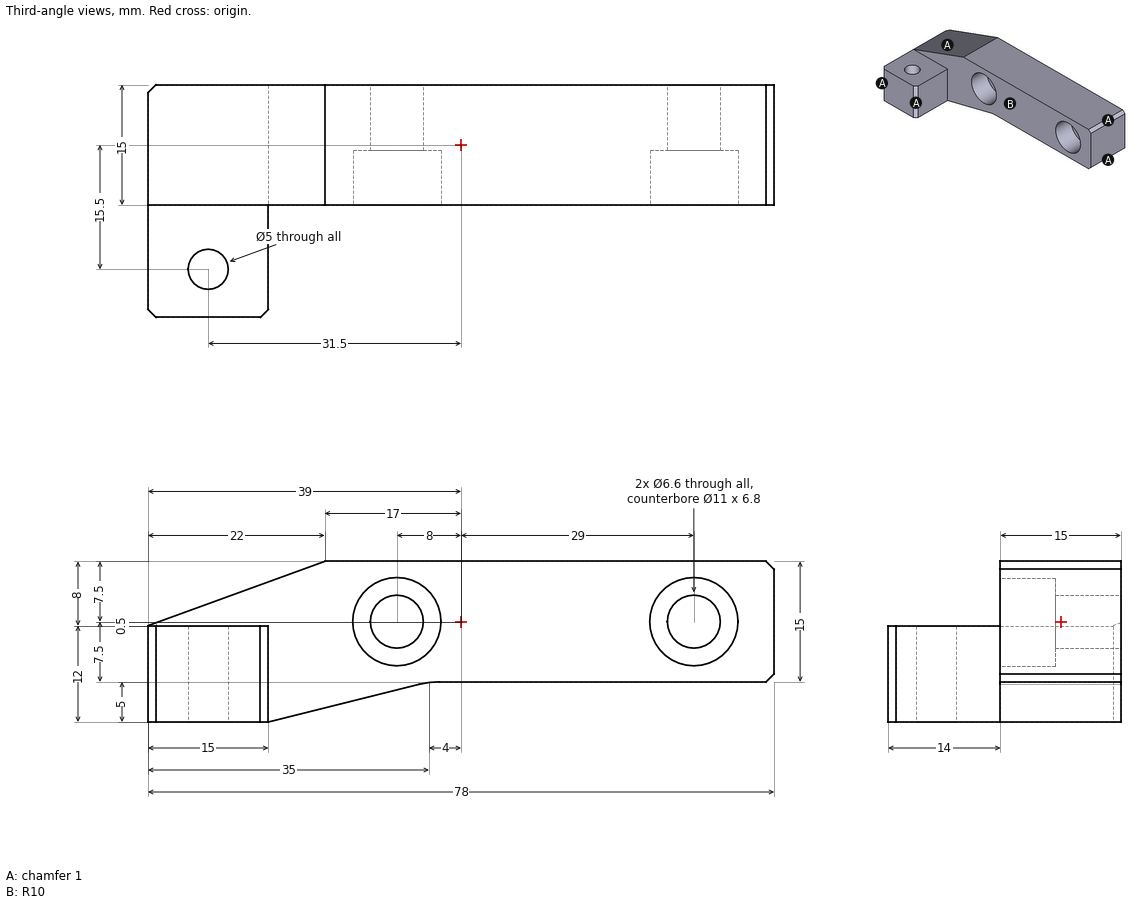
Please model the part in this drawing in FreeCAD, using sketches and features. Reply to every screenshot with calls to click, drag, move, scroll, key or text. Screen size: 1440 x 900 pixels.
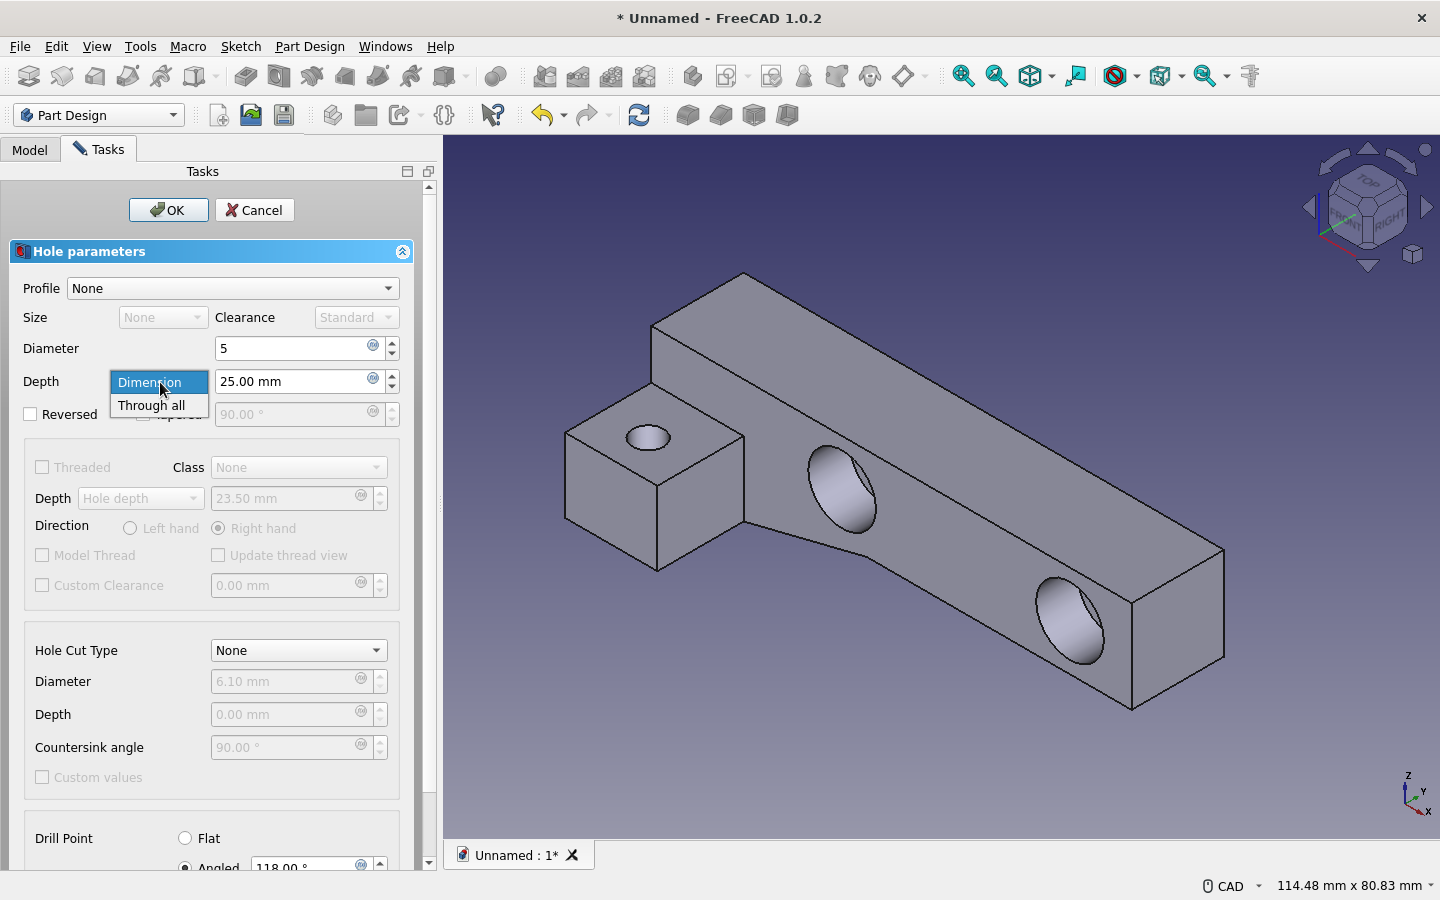
click(158, 406)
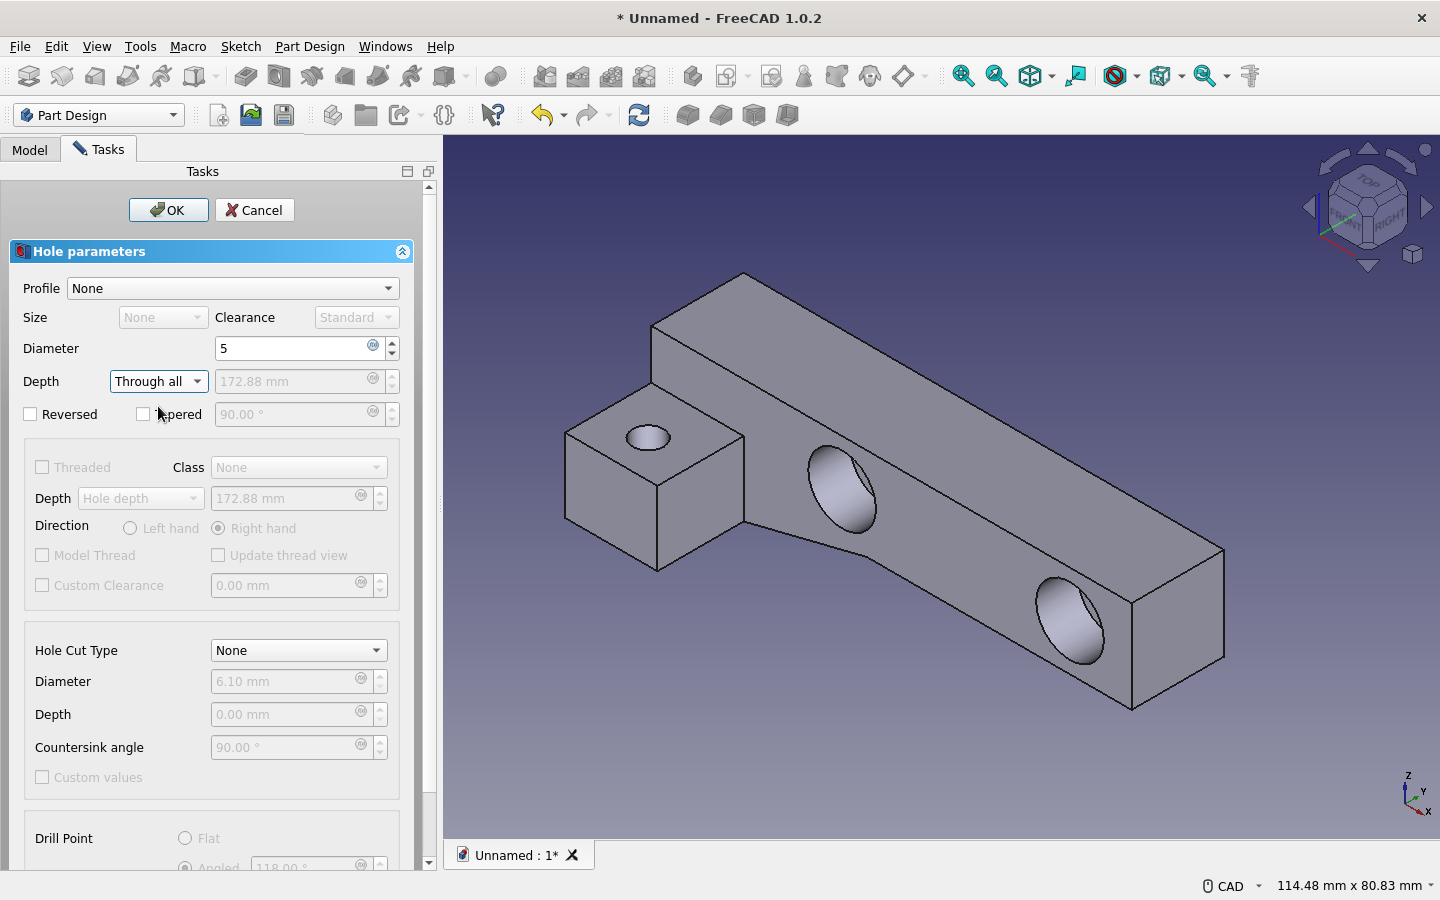
click(169, 210)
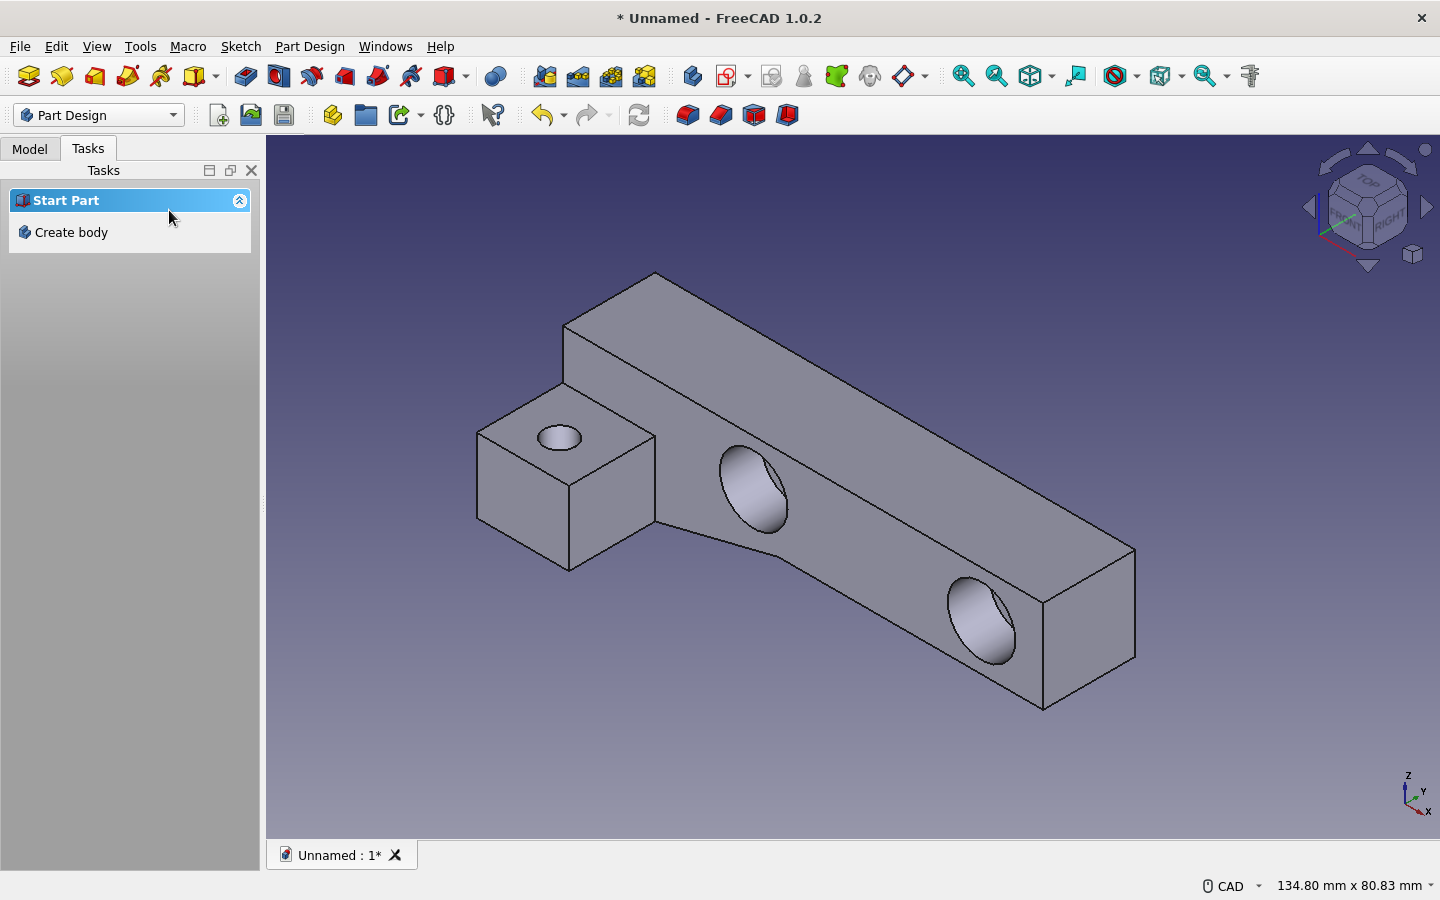
click(523, 501)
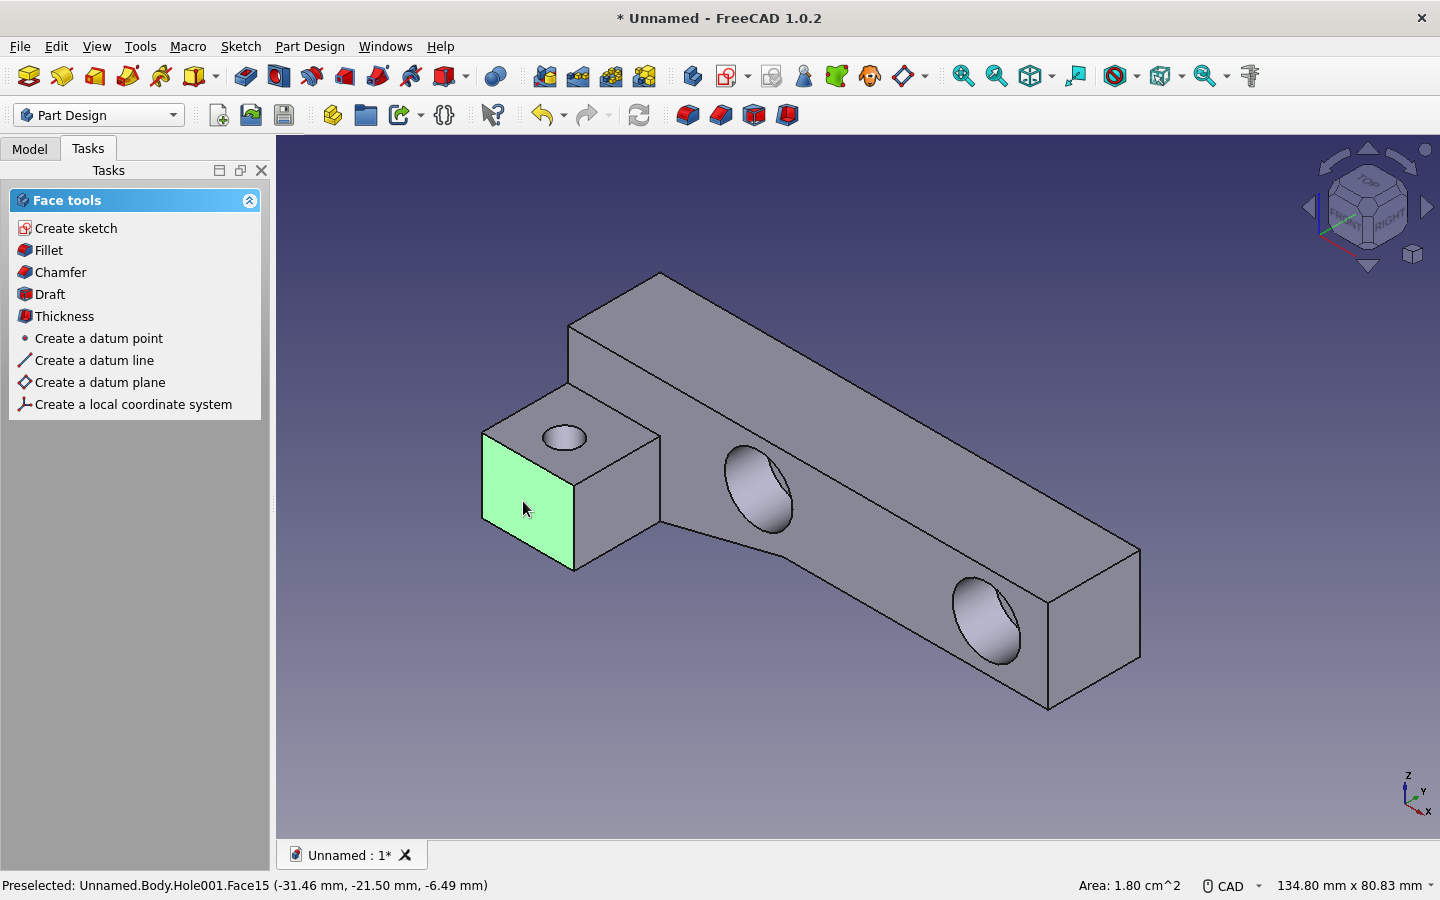
click(726, 76)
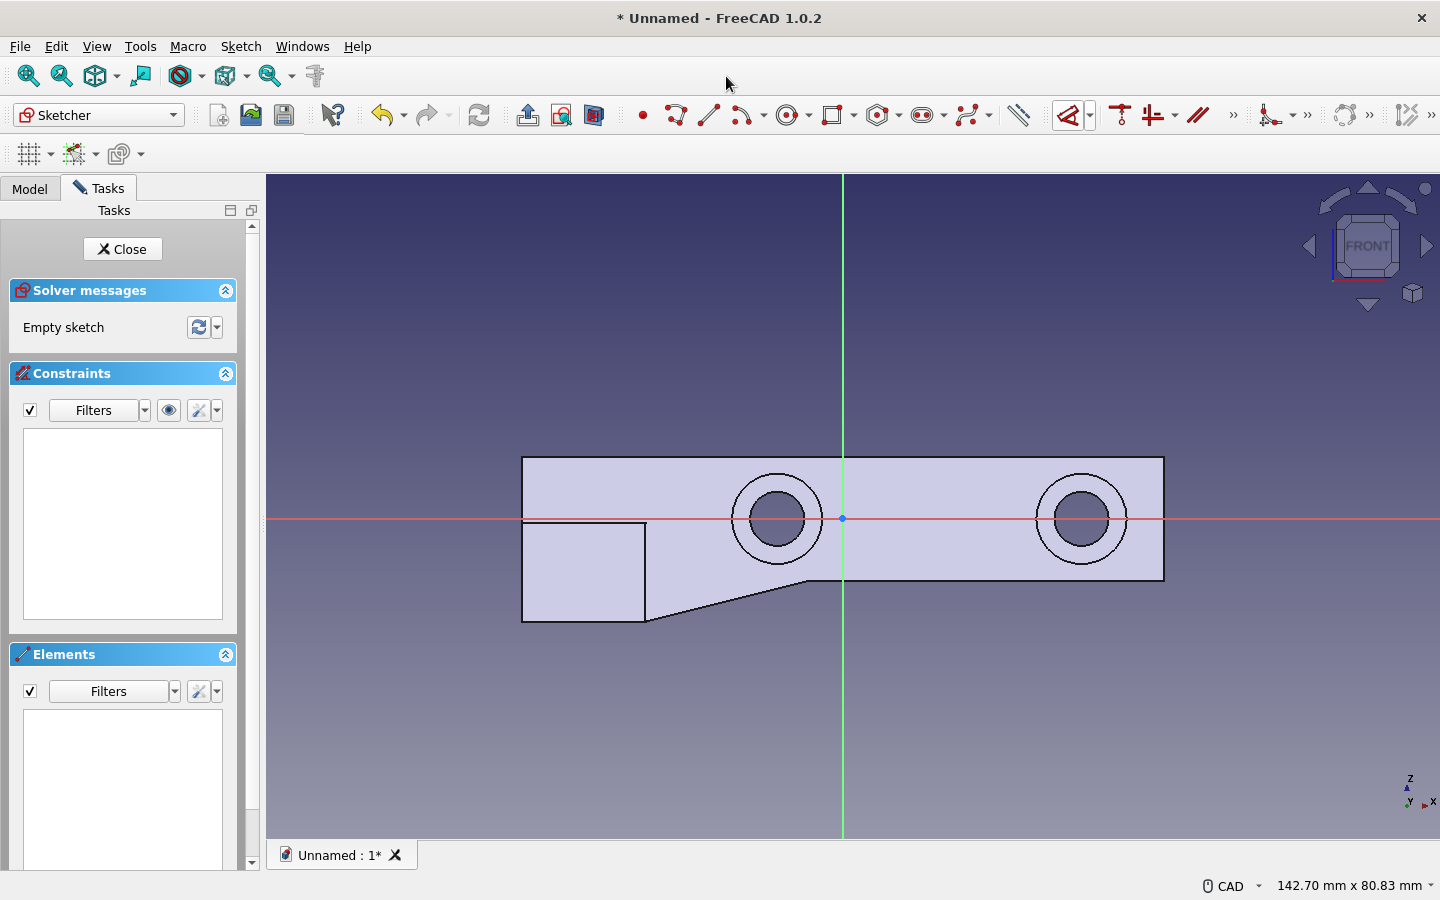
scroll(599, 477, up, 4)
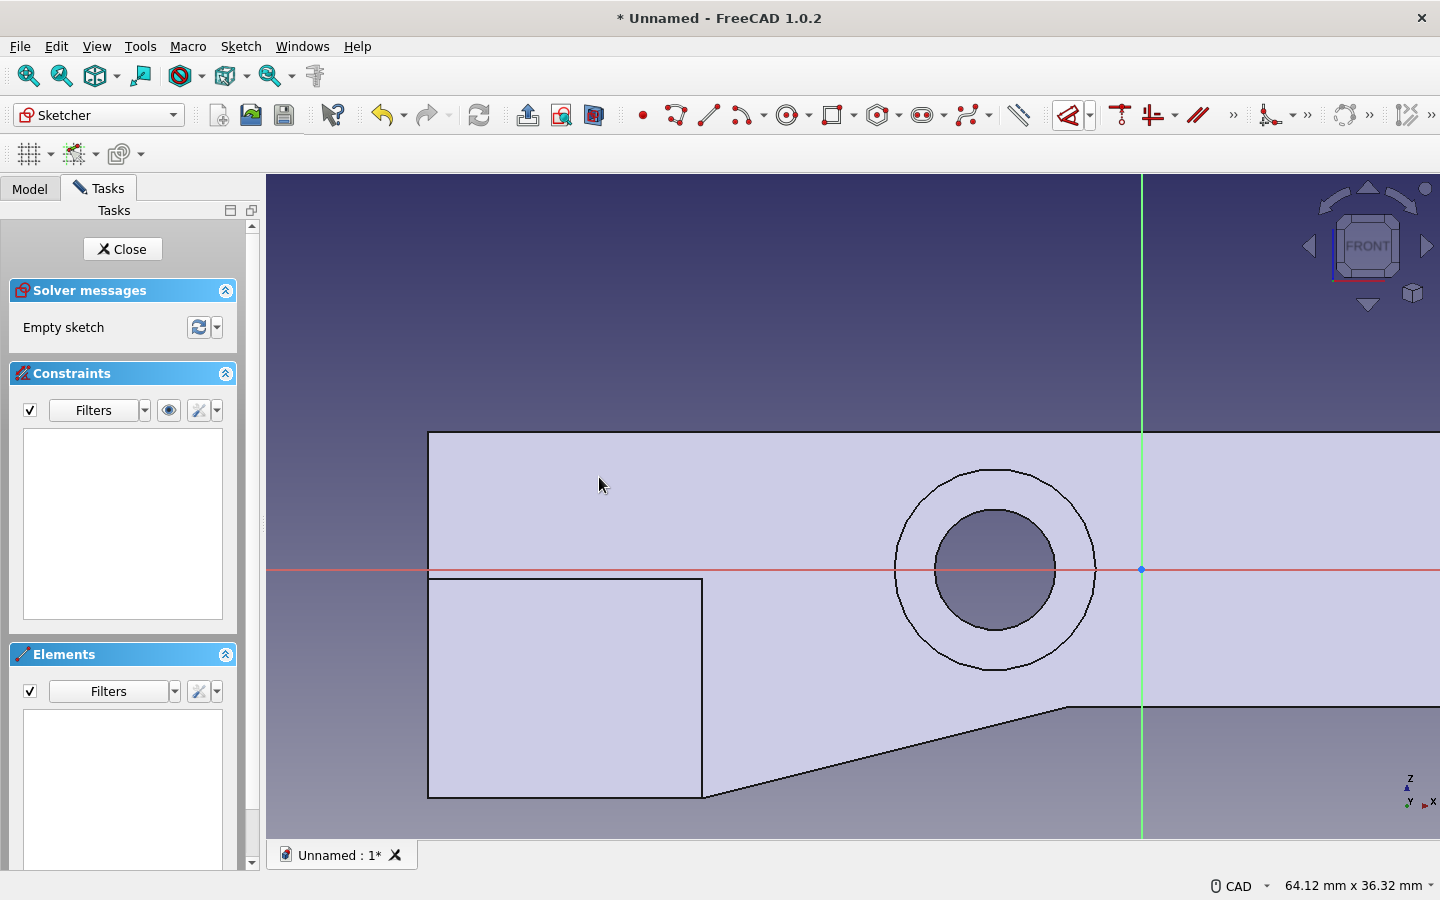
click(676, 116)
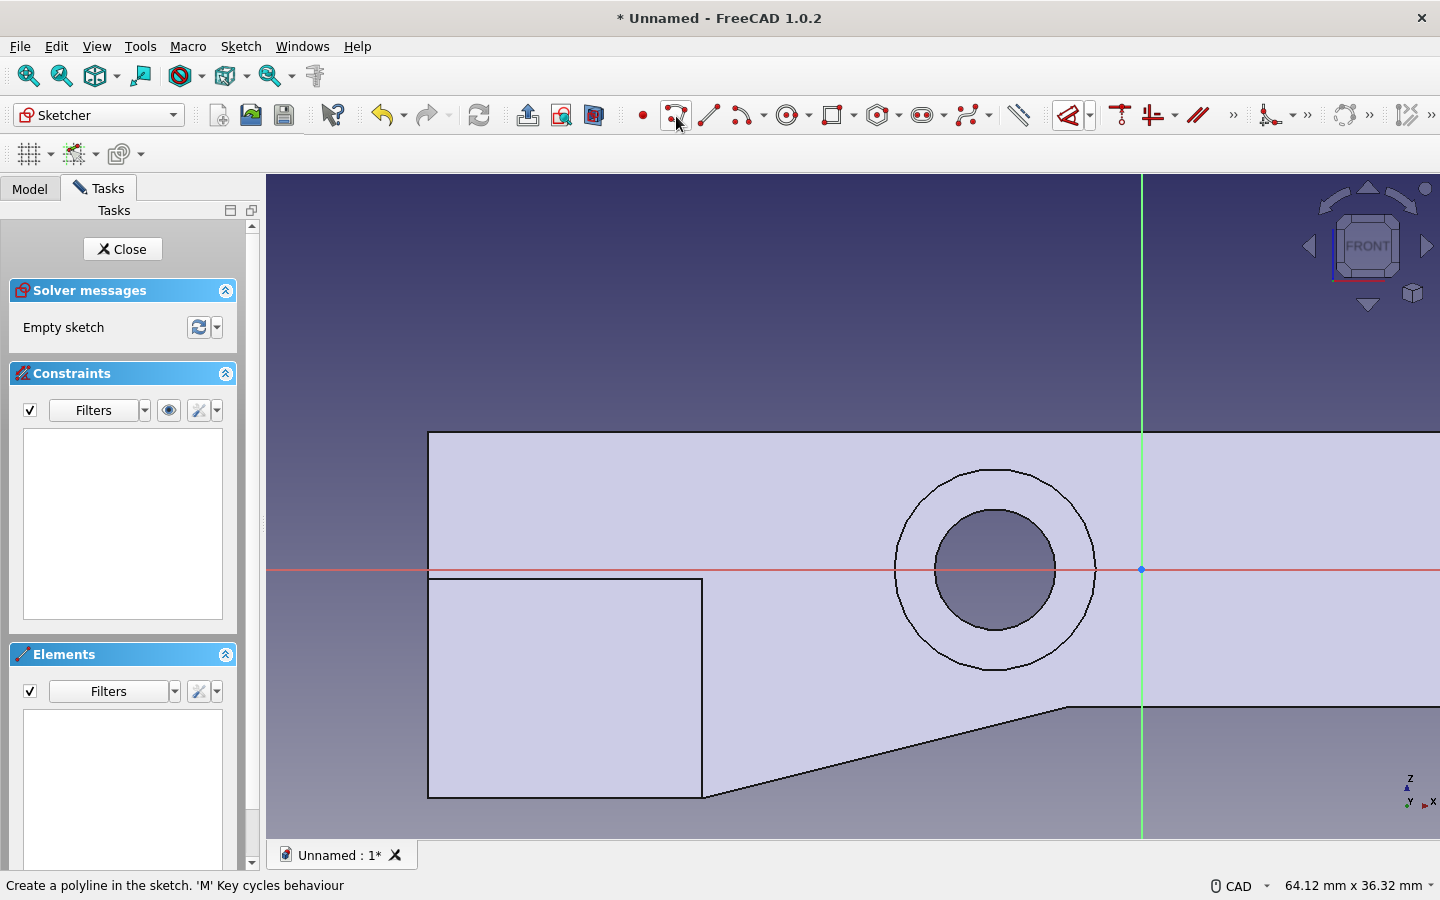
click(830, 432)
click(428, 432)